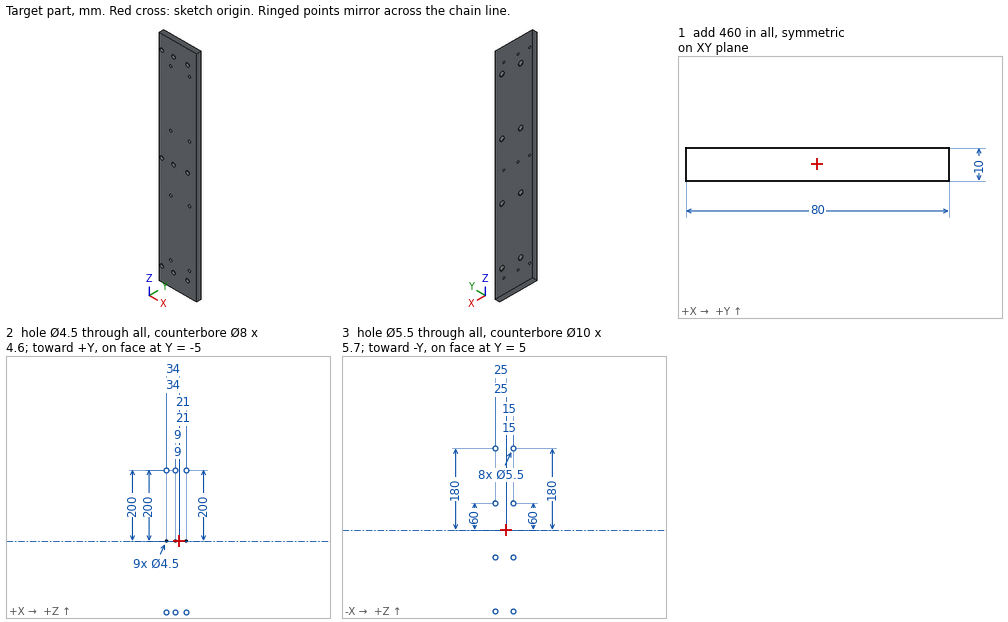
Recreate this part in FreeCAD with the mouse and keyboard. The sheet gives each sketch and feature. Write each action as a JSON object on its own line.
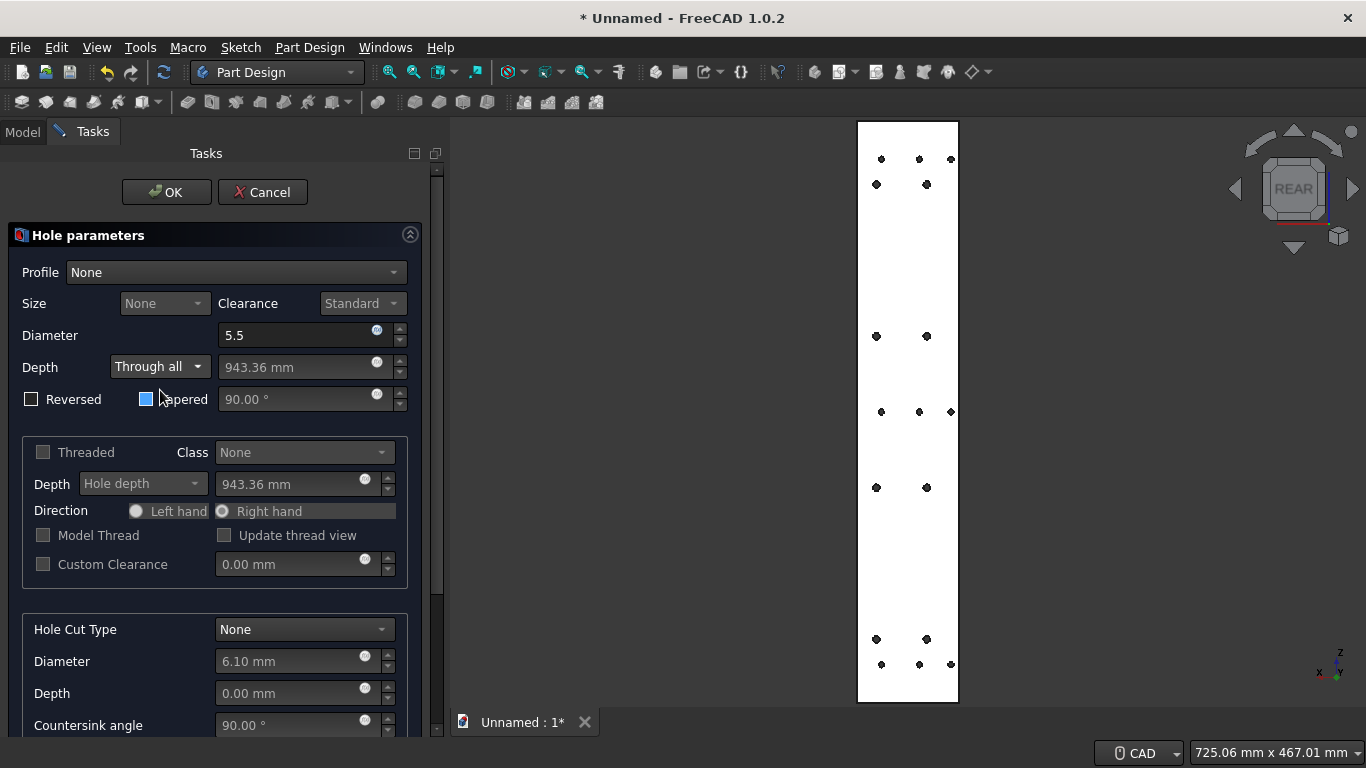
{"action": "left_click", "coordinate": [306, 630]}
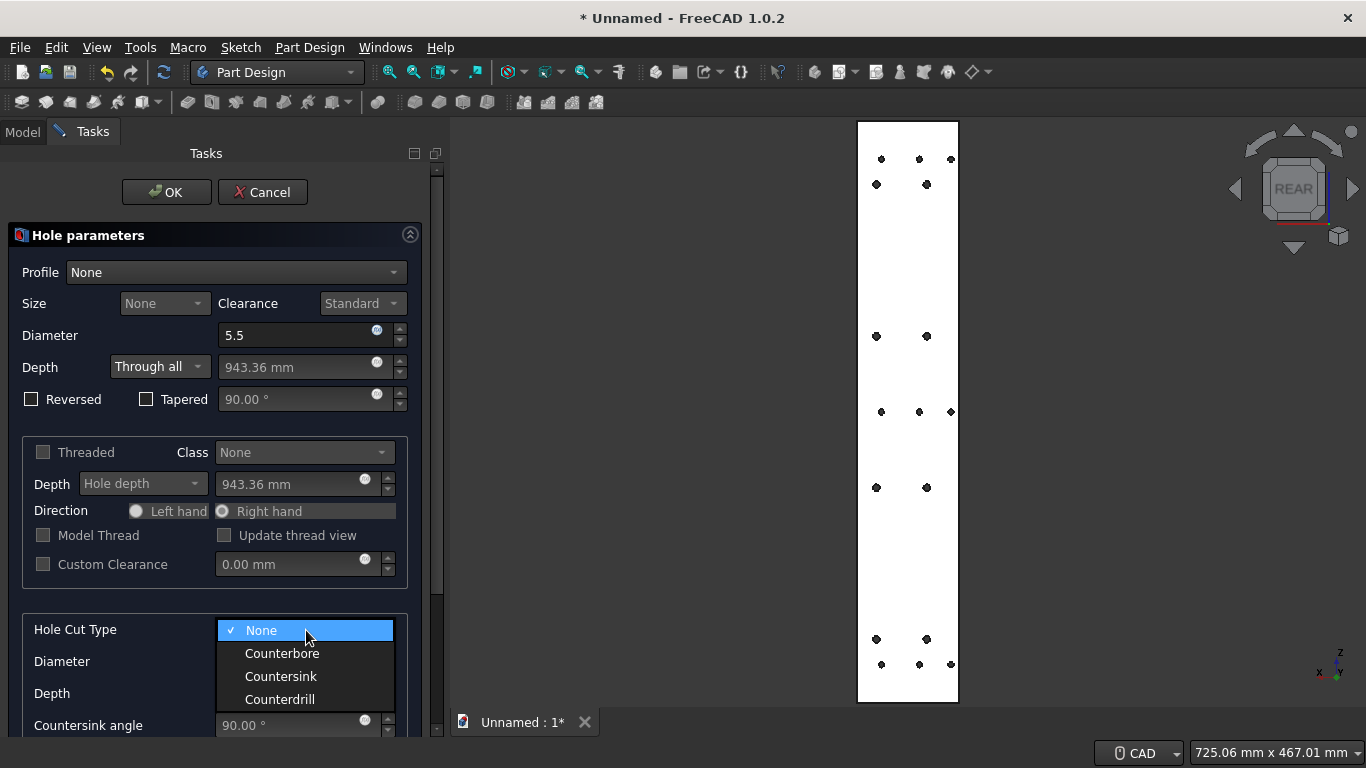
{"action": "left_click", "coordinate": [304, 654]}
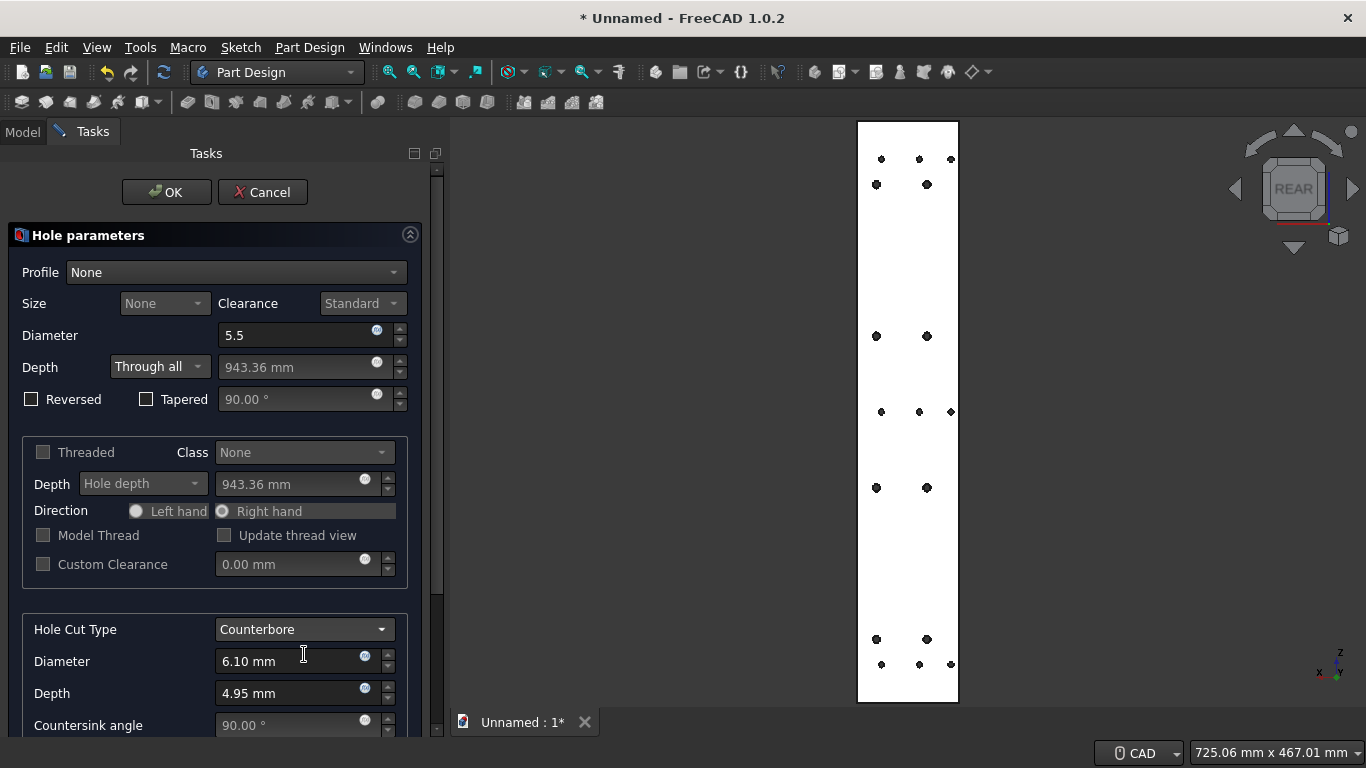
{"action": "triple_click", "coordinate": [298, 661]}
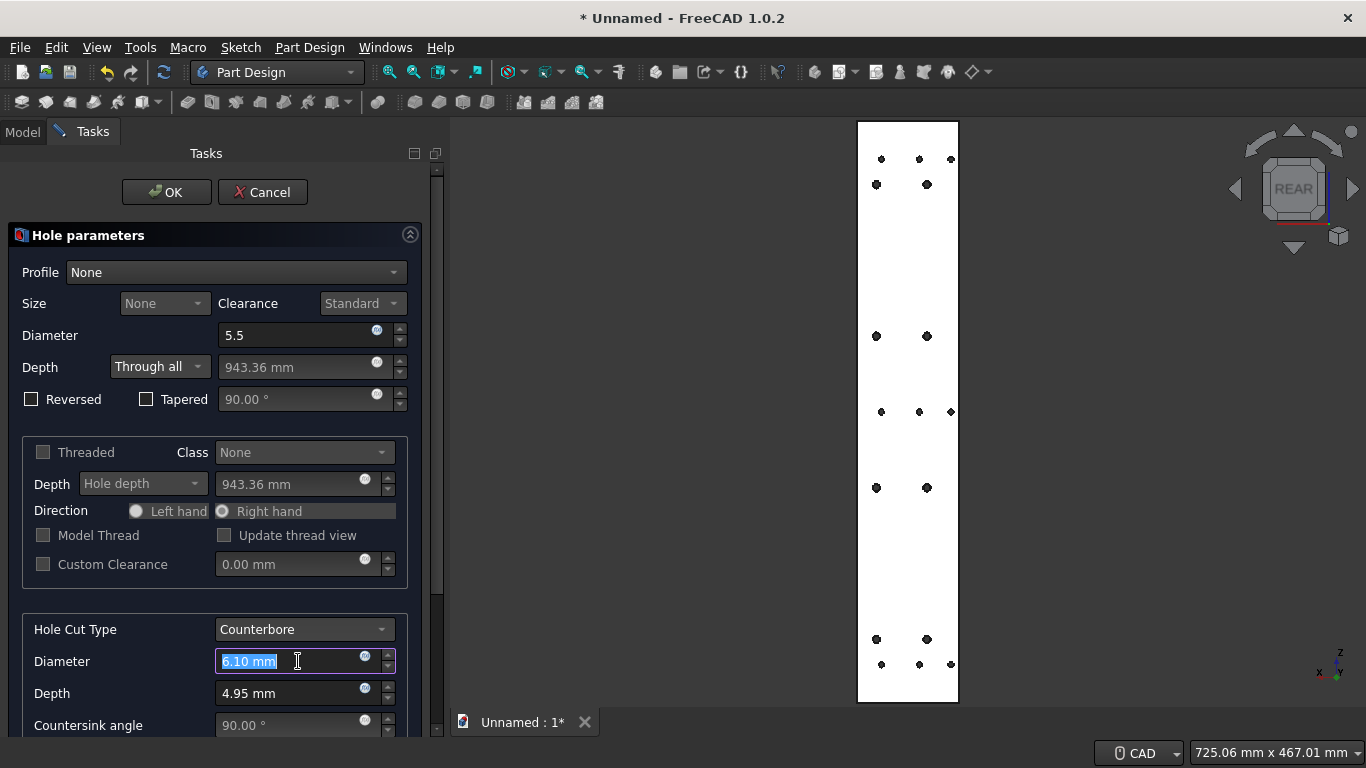
{"action": "type", "text": "10"}
{"action": "key", "text": "Tab"}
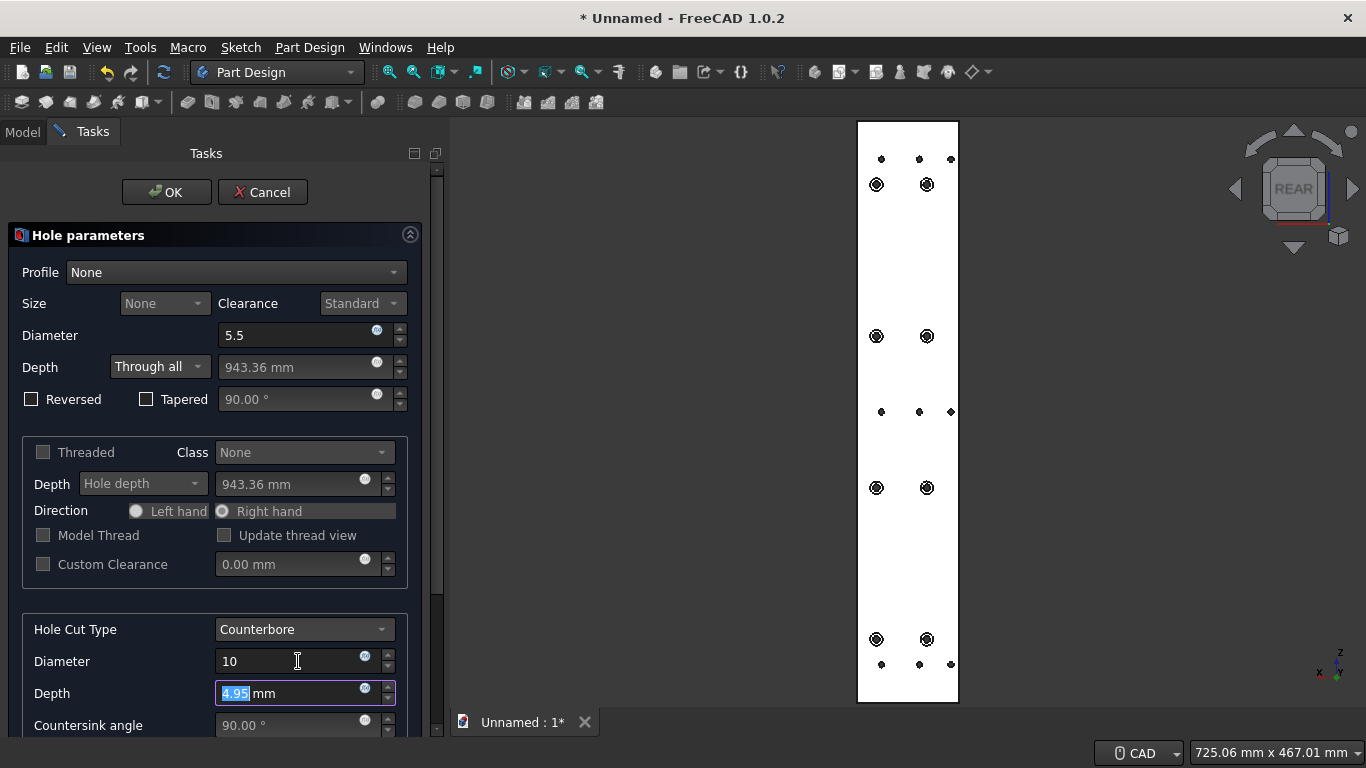
{"action": "type", "text": "5.7"}
{"action": "key", "text": "Tab"}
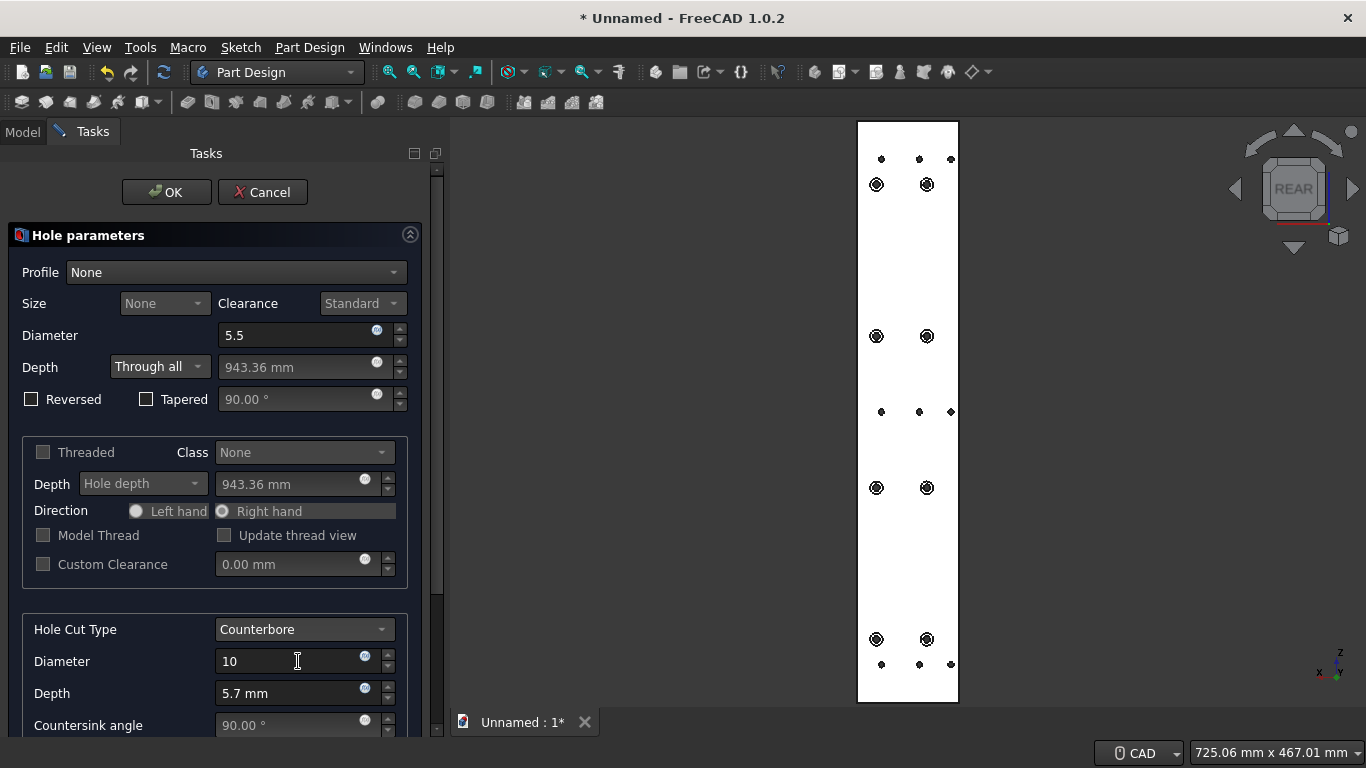
{"action": "left_click", "coordinate": [167, 192]}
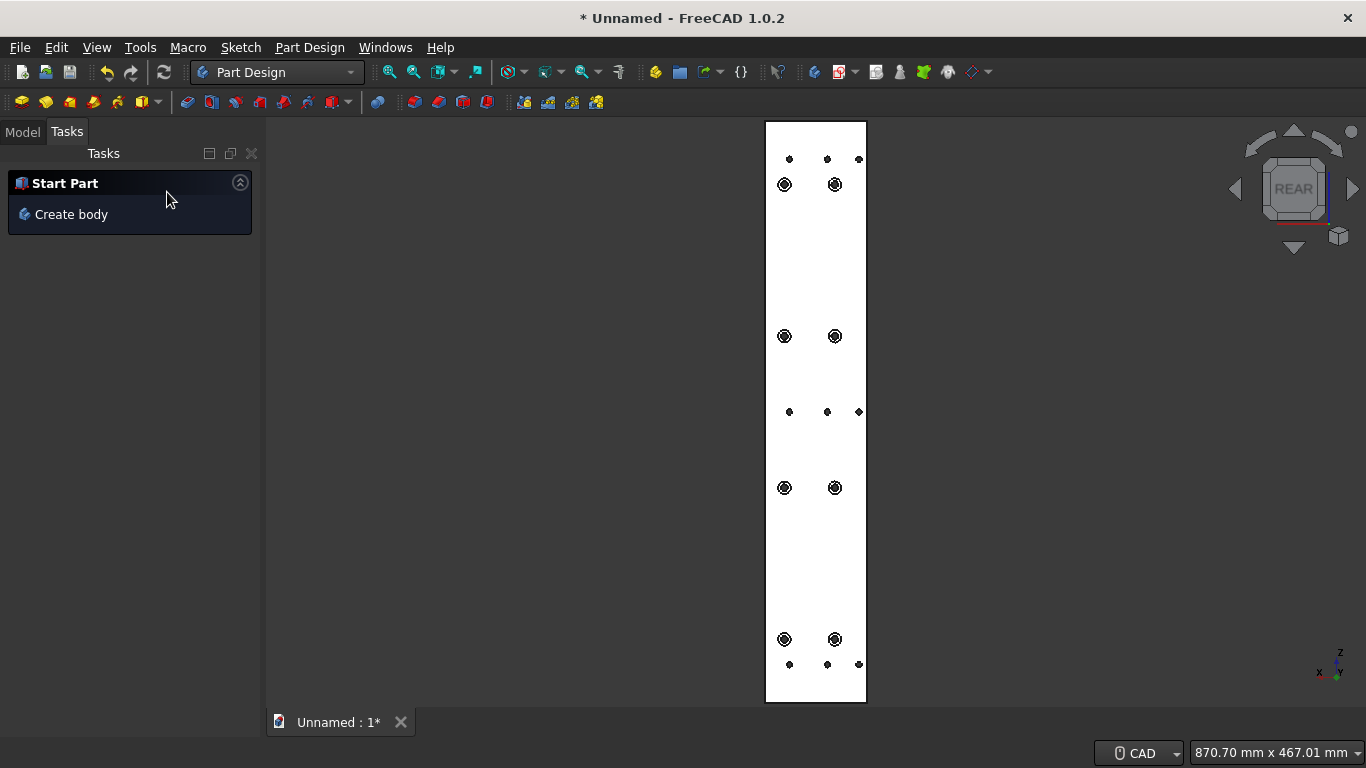
{"action": "key", "text": "0"}